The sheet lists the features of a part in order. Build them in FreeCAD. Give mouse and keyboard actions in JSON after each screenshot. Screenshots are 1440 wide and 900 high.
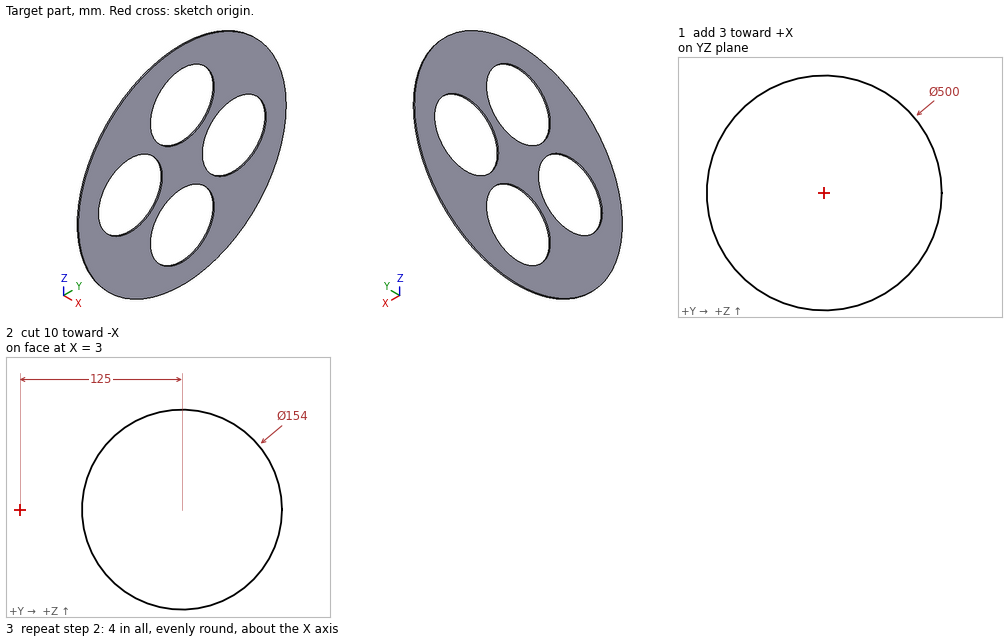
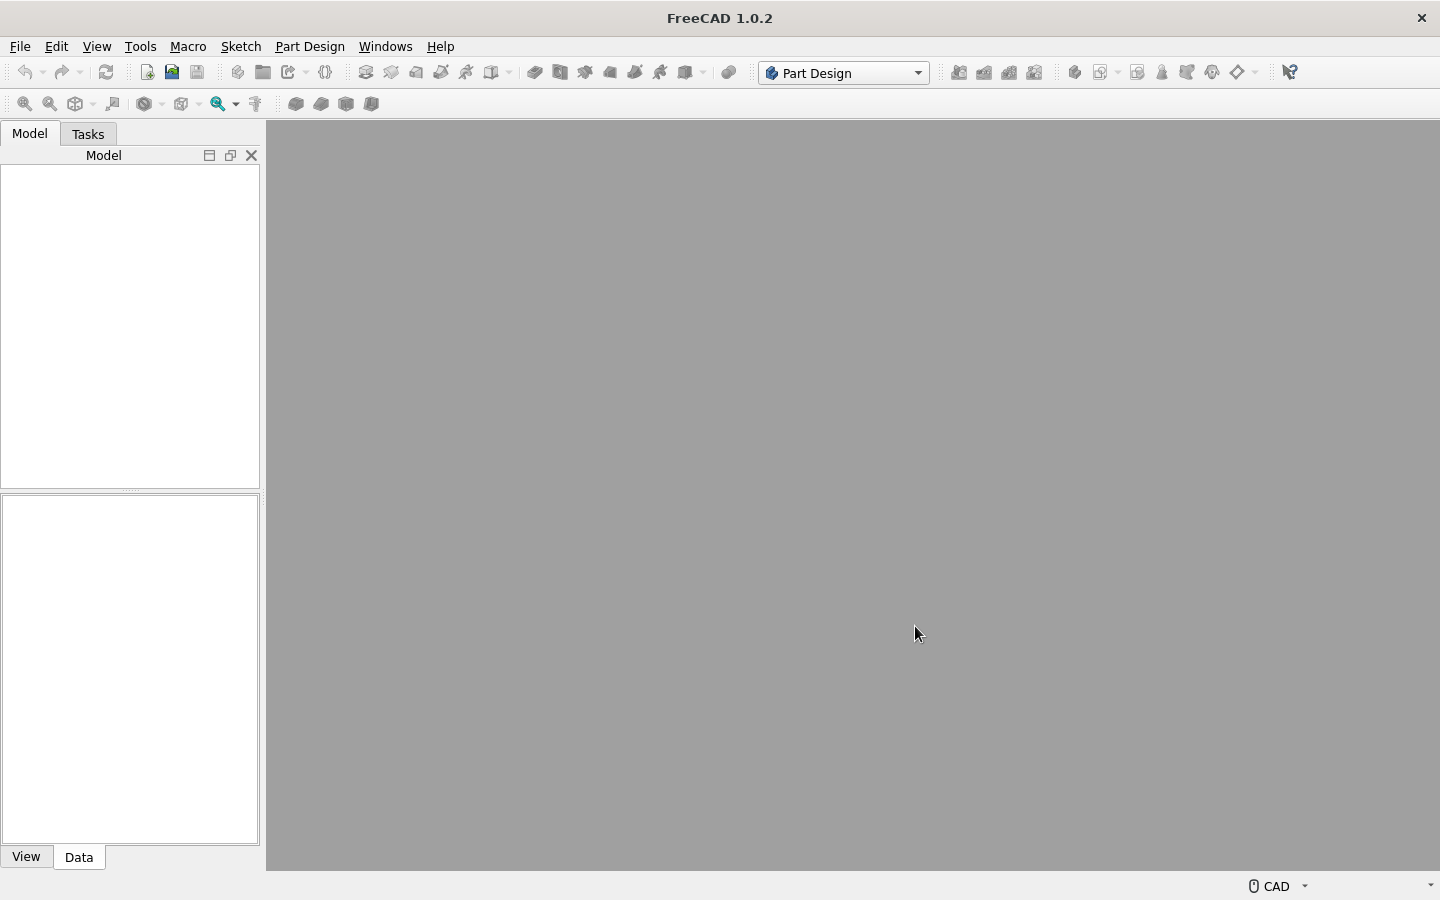
{"action": "left_click", "coordinate": [147, 72]}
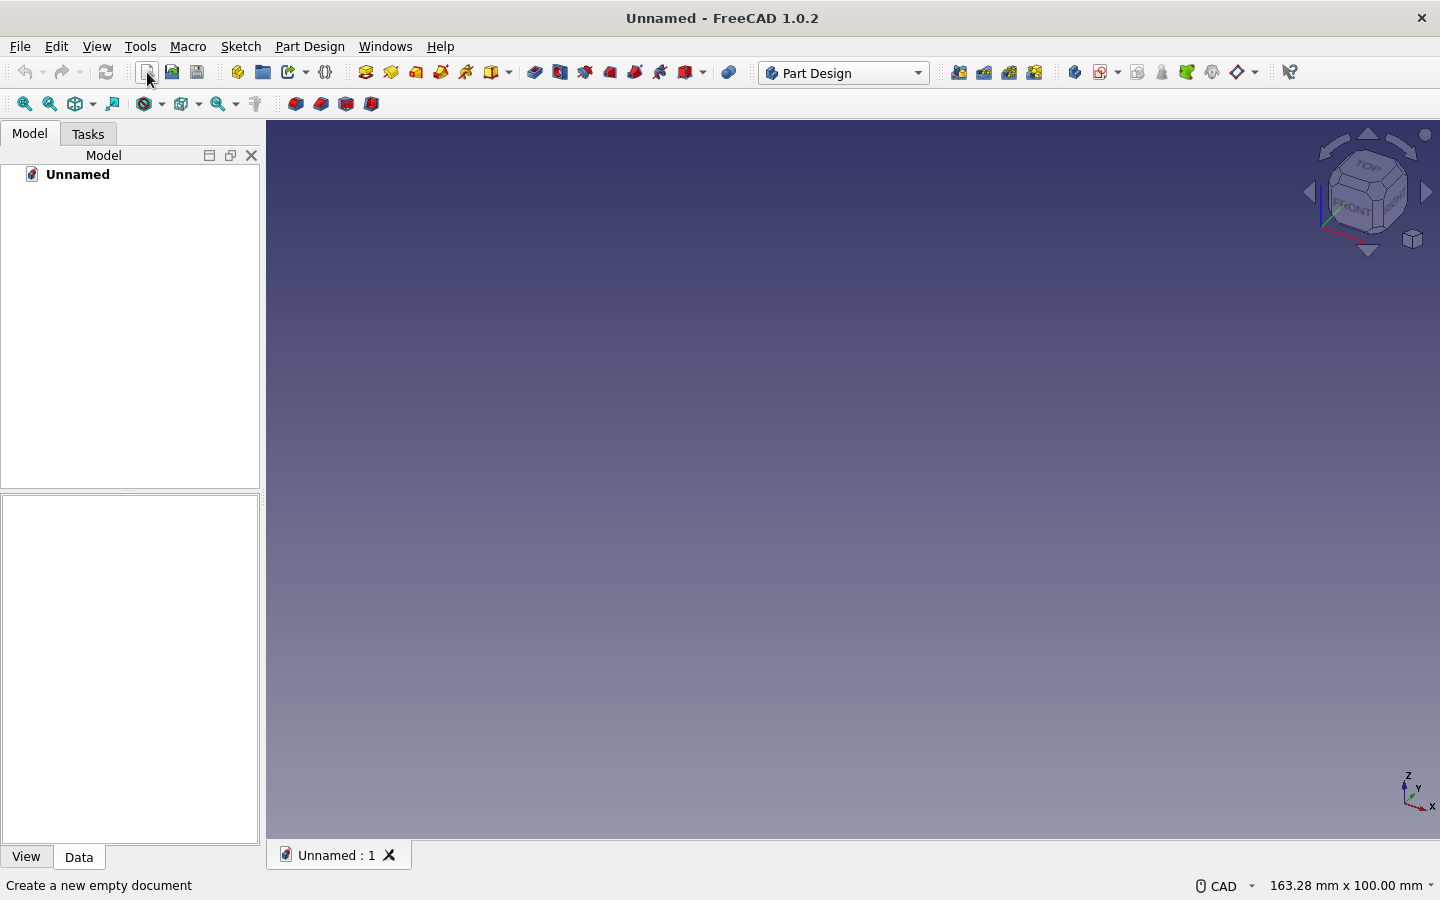
{"action": "left_click", "coordinate": [1100, 72]}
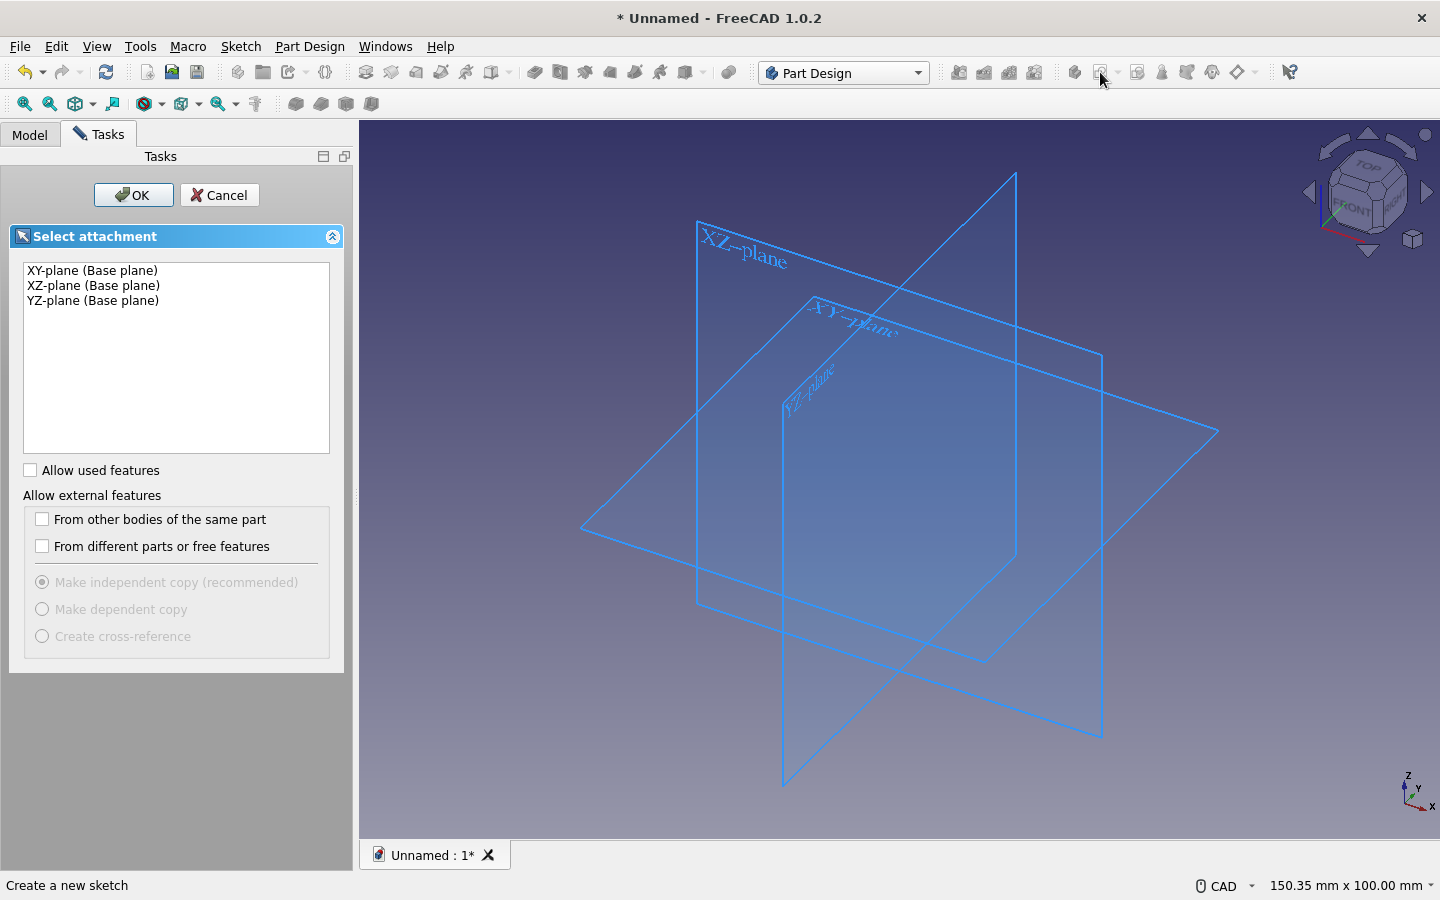
{"action": "left_click", "coordinate": [84, 300]}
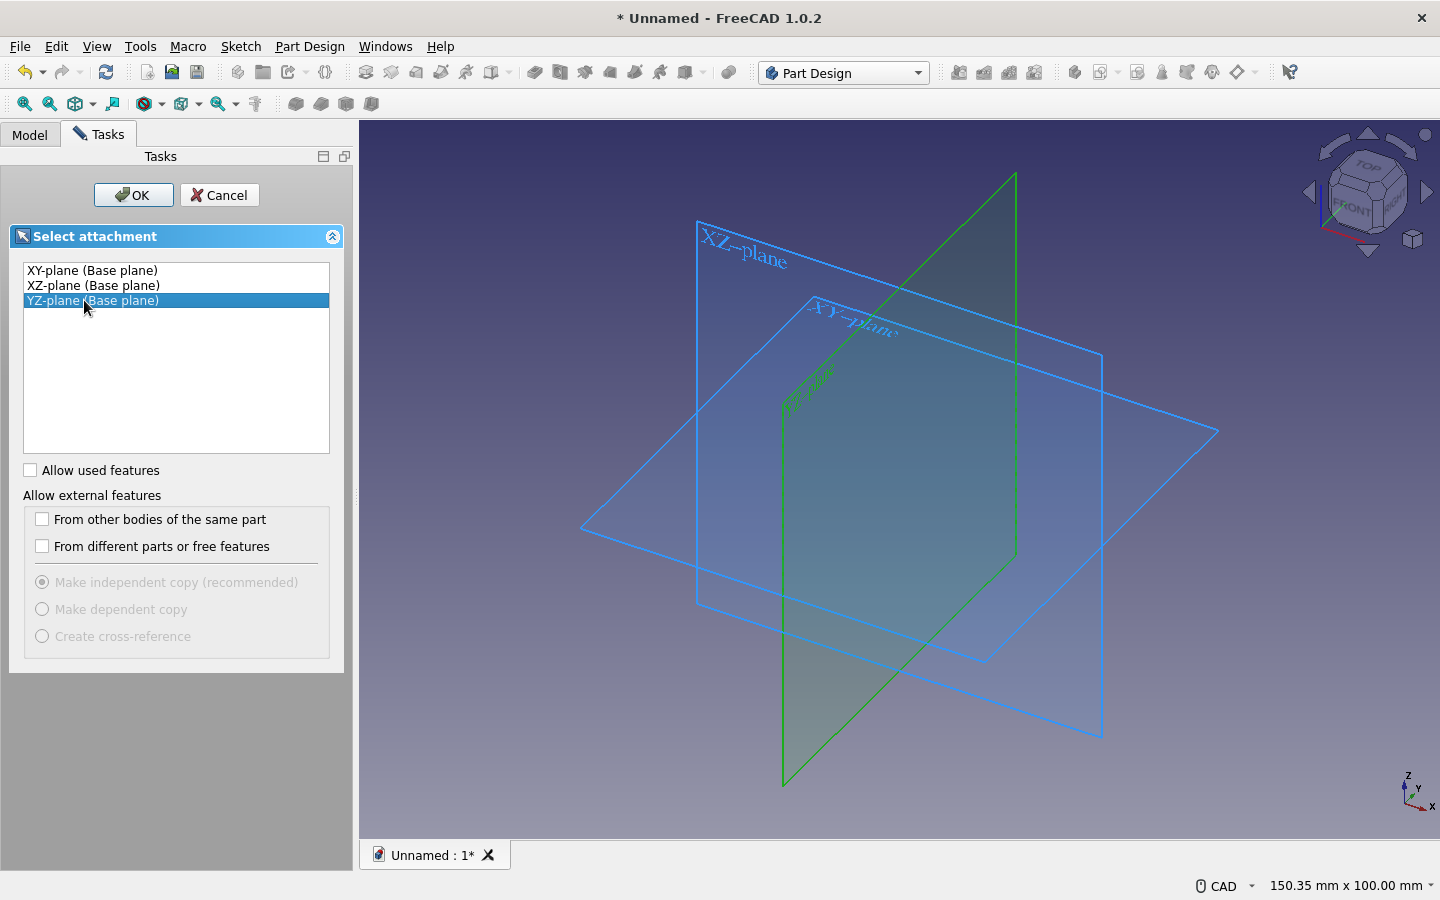
{"action": "left_click", "coordinate": [134, 195]}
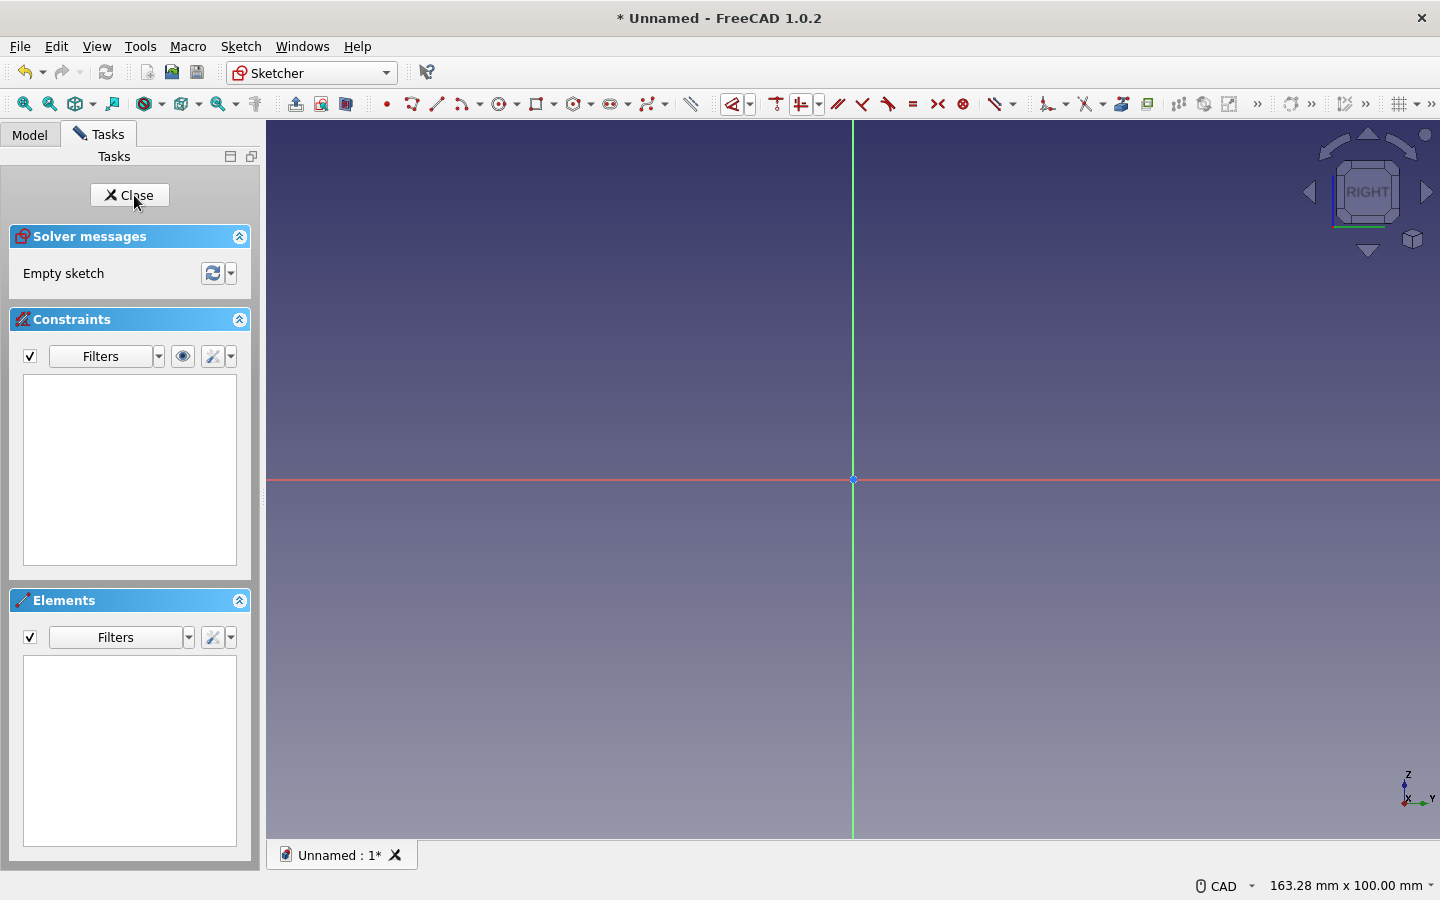
{"action": "scroll", "coordinate": [774, 480], "scroll_direction": "down", "scroll_amount": 10}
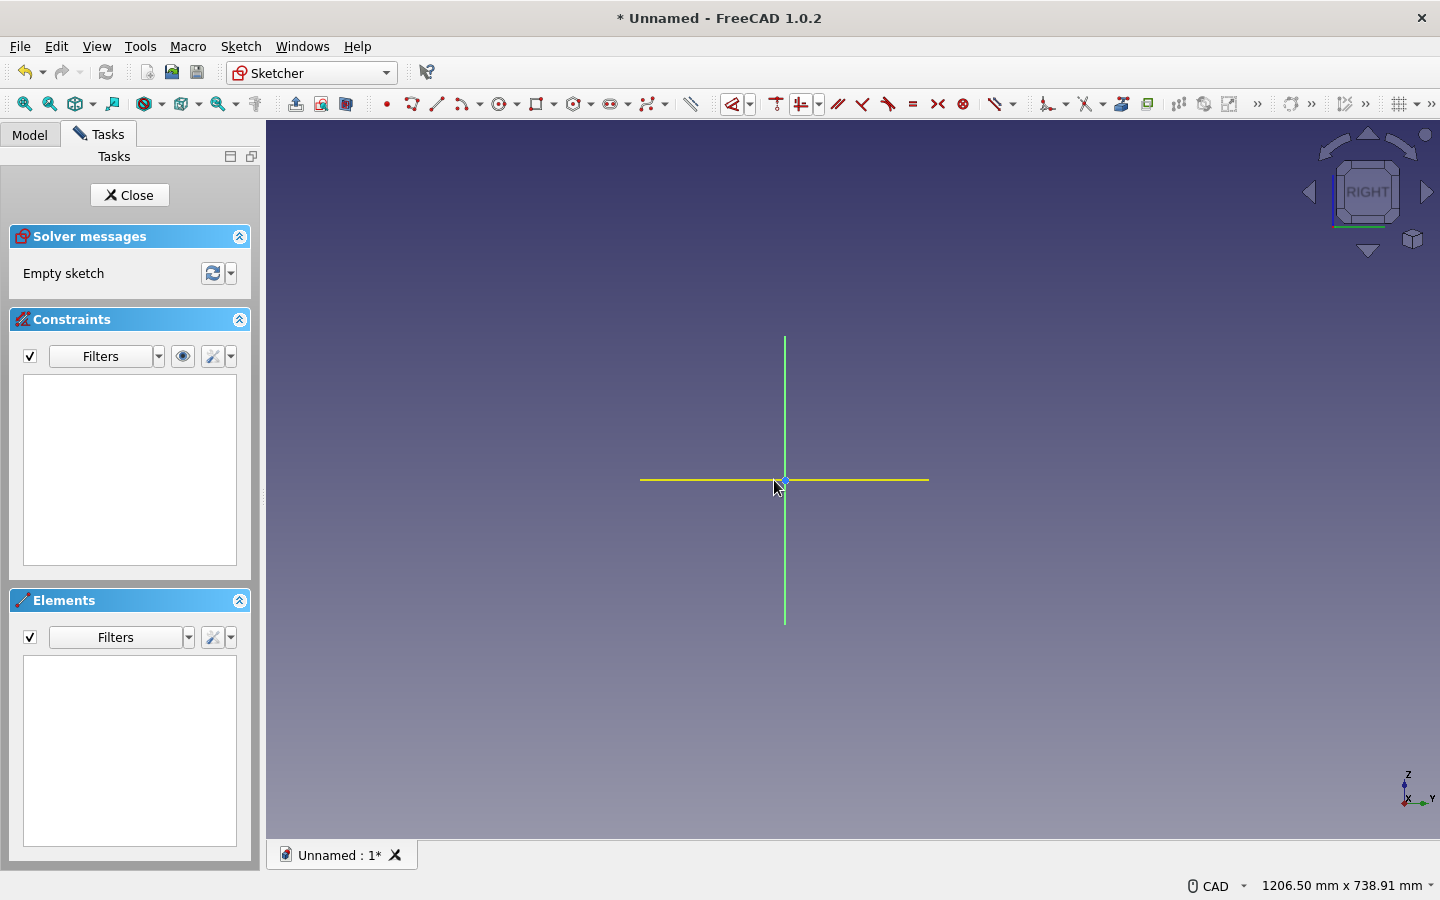
{"action": "left_click", "coordinate": [498, 104]}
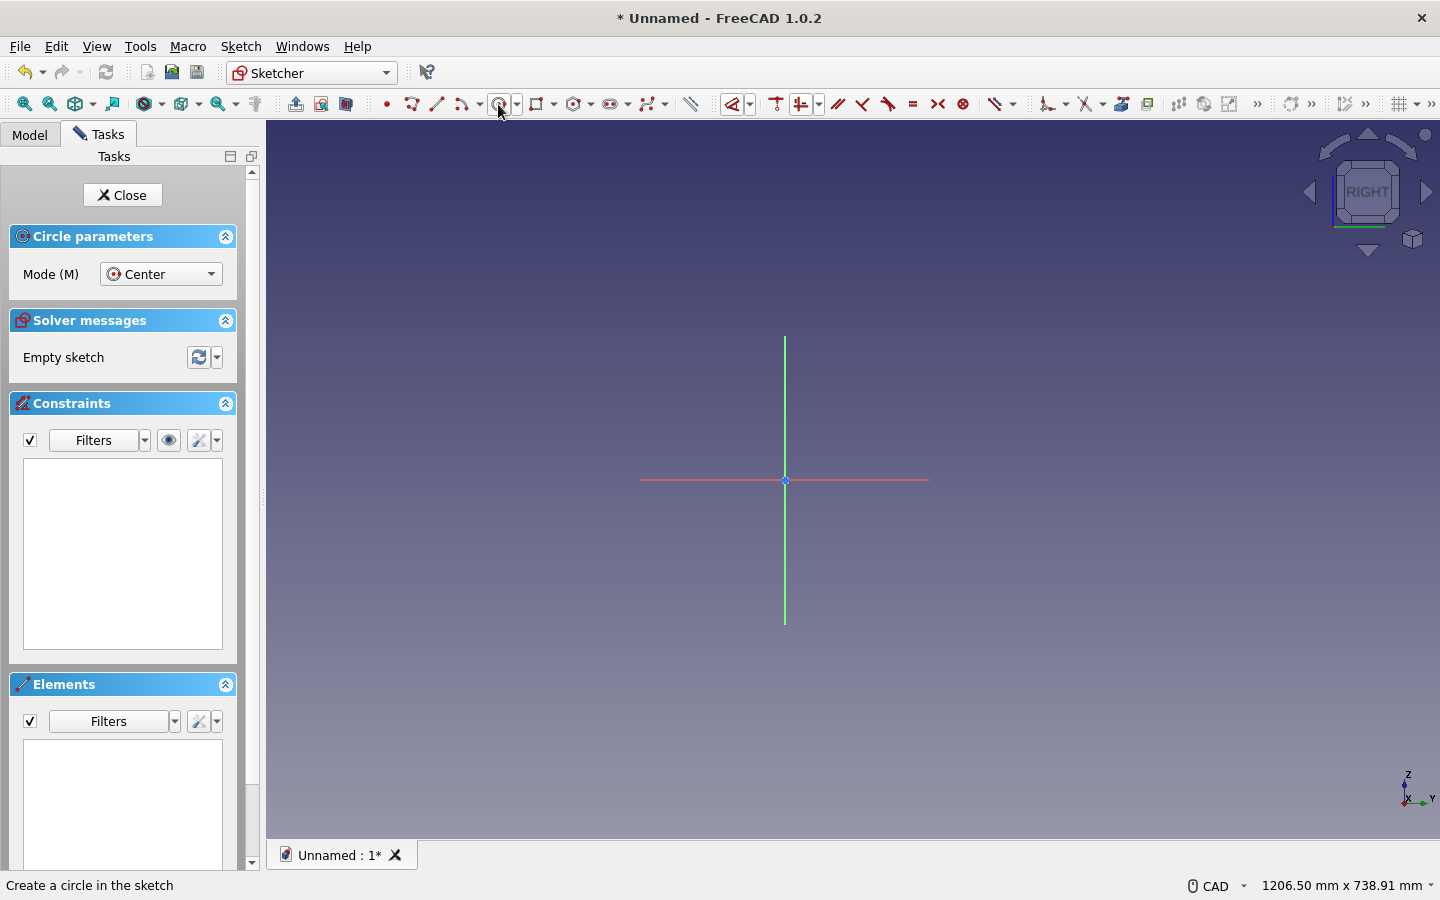
{"action": "left_click", "coordinate": [785, 480]}
{"action": "left_click", "coordinate": [957, 308]}
{"action": "key", "text": "Escape"}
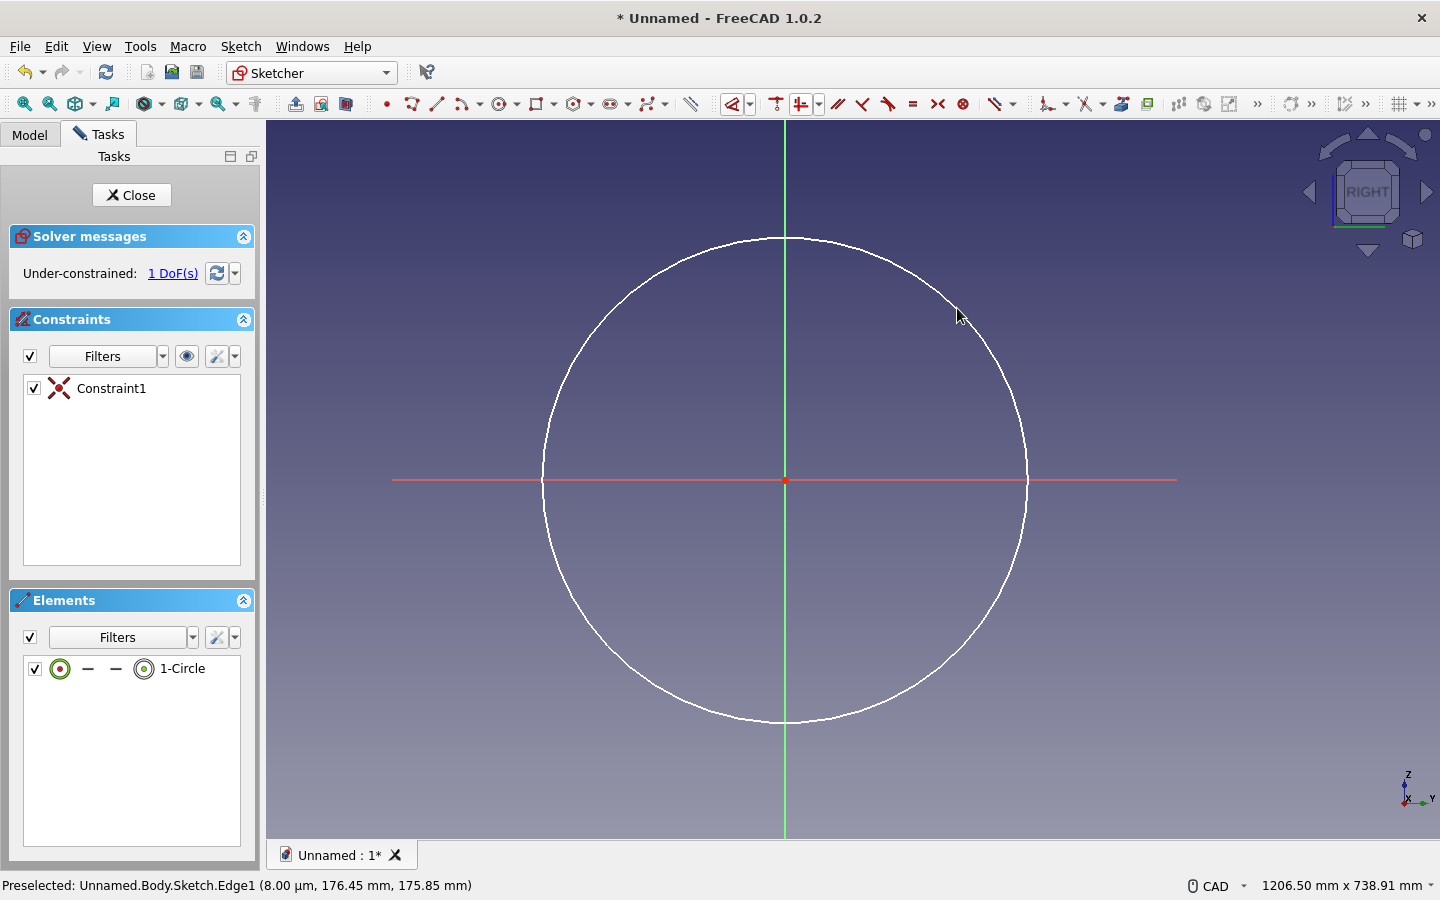
{"action": "left_click", "coordinate": [732, 104]}